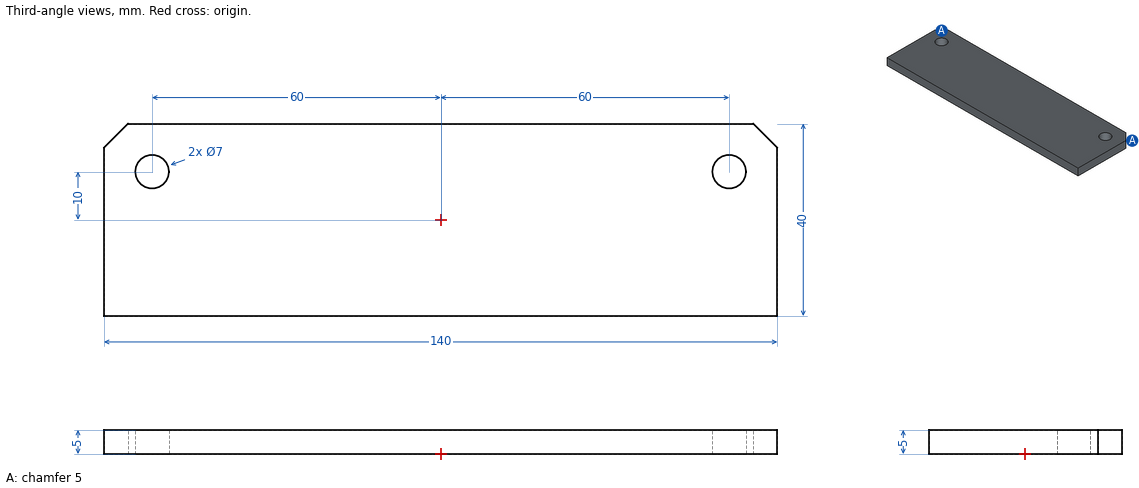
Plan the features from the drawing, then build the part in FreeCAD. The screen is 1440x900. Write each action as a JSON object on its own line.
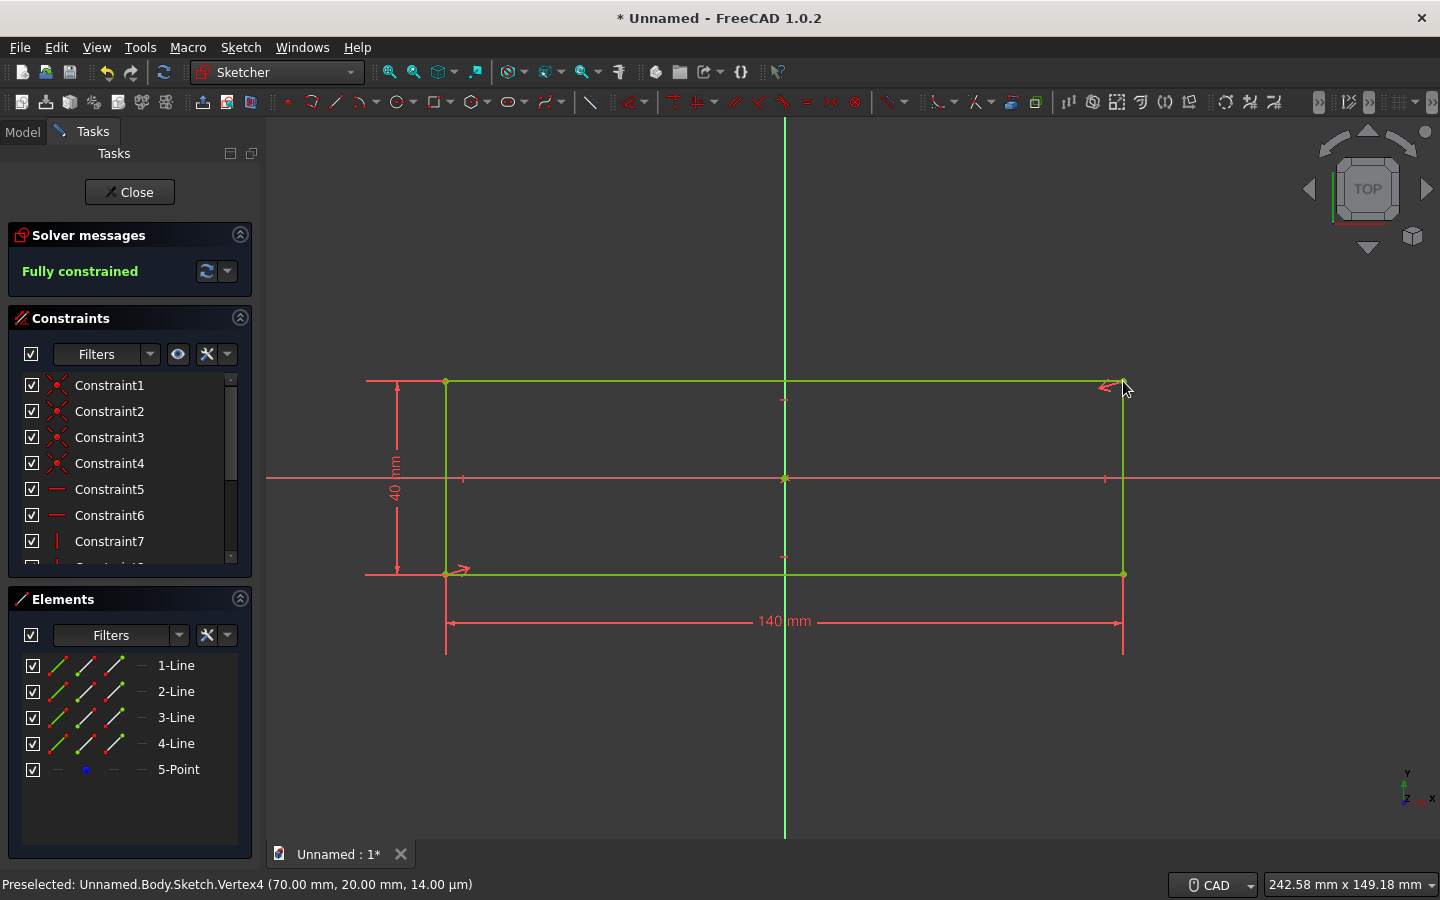
{"action": "left_click", "coordinate": [130, 192]}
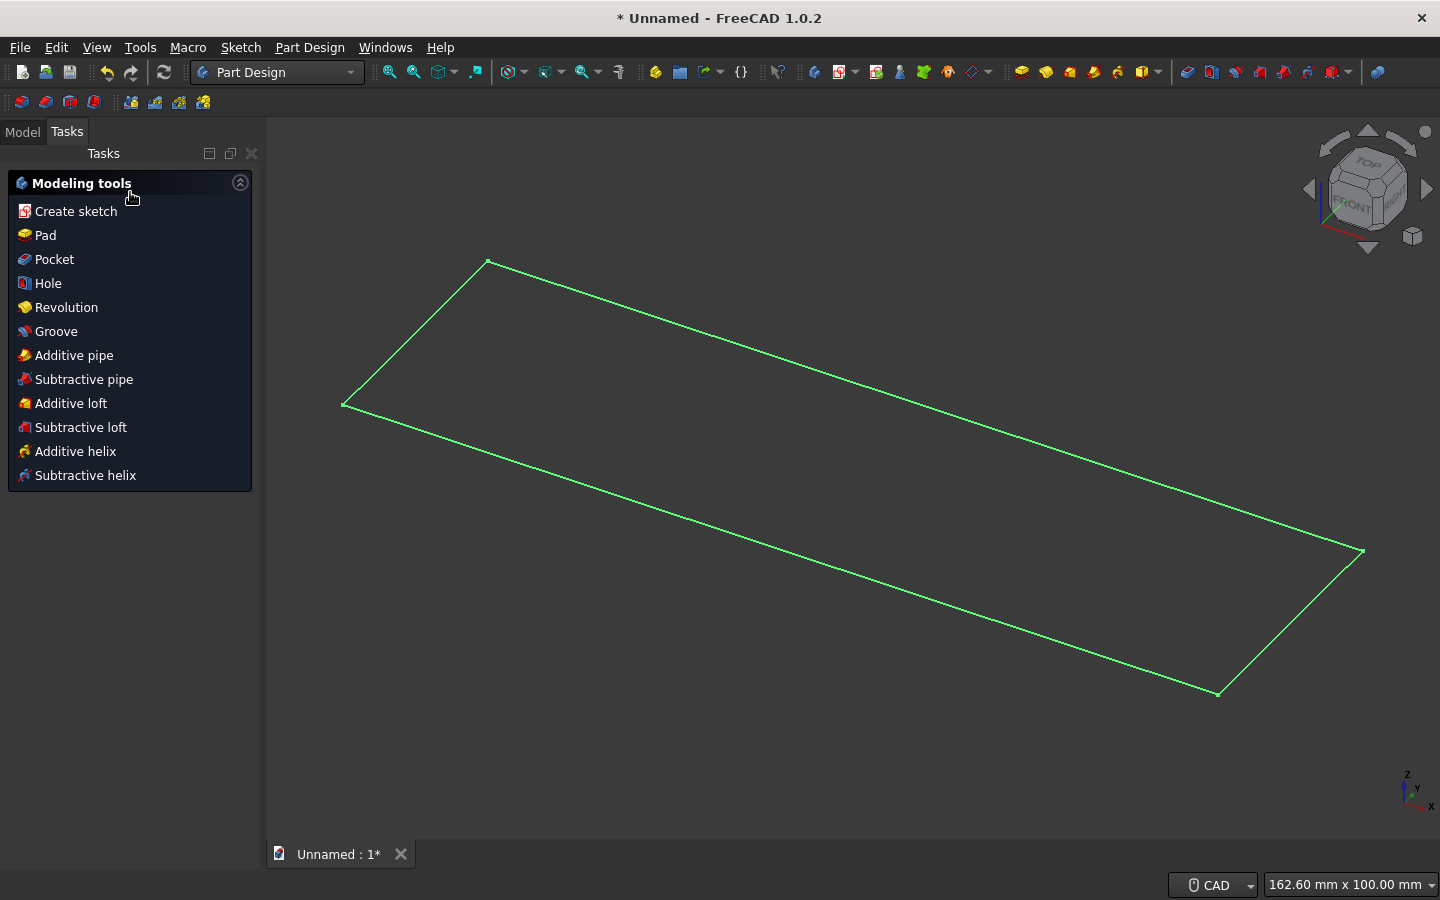
{"action": "left_click", "coordinate": [1022, 72]}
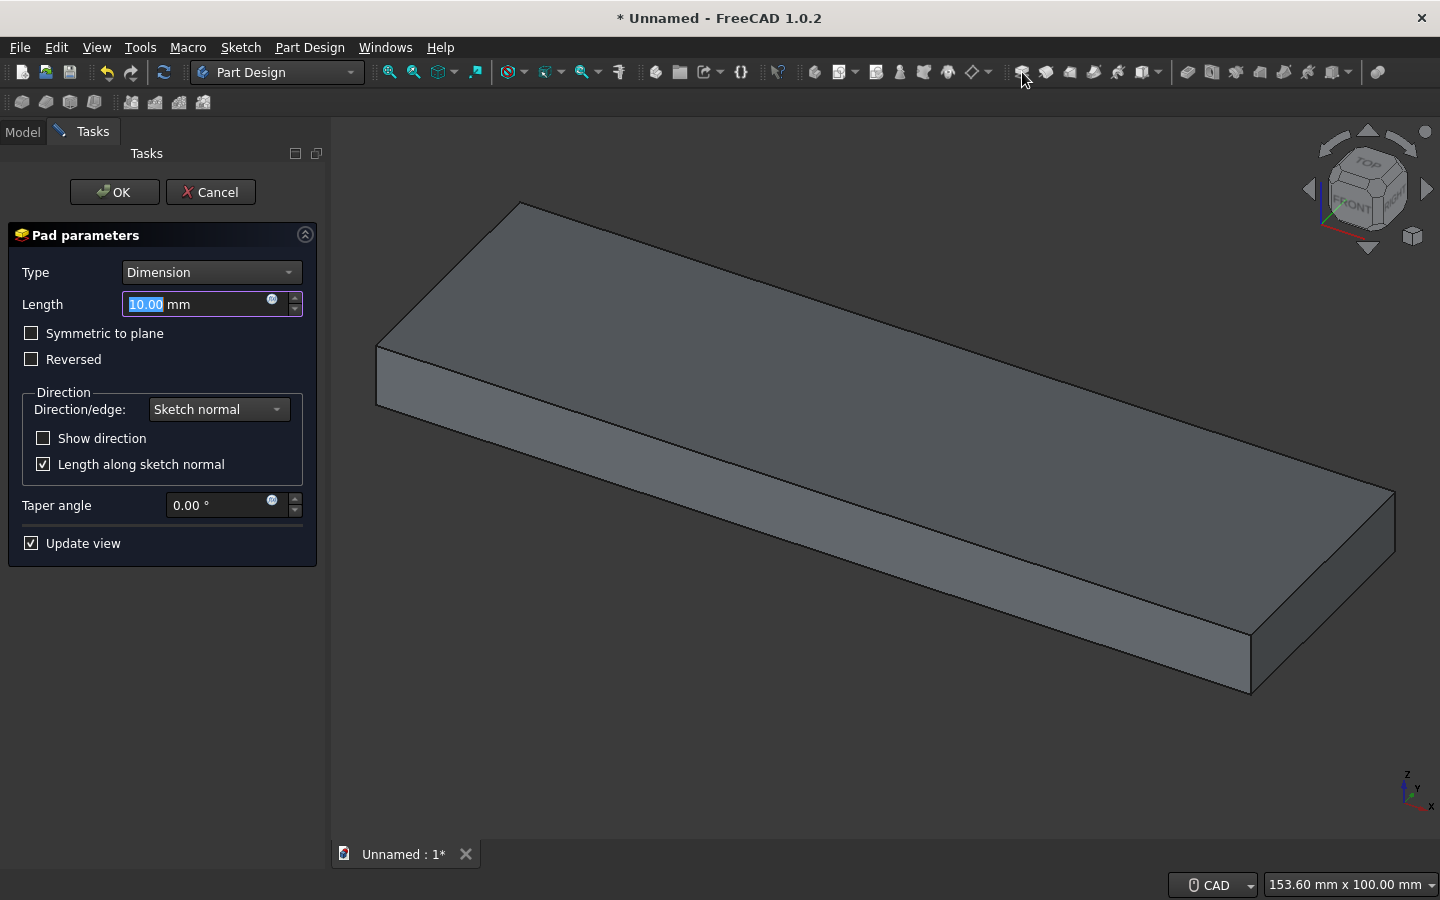
{"action": "type", "text": "5"}
{"action": "key", "text": "Tab"}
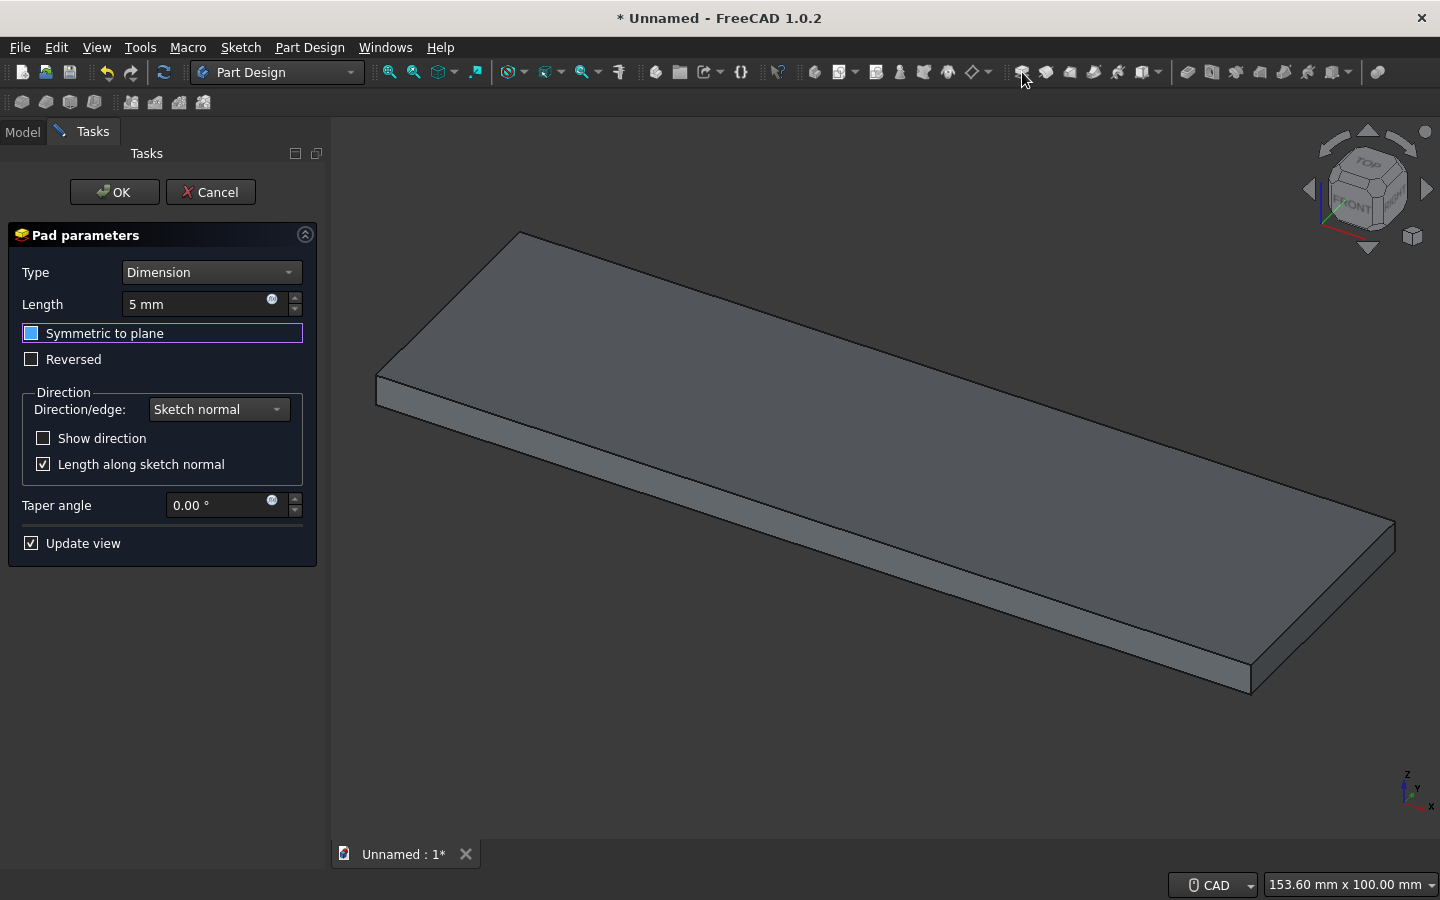
{"action": "left_click", "coordinate": [115, 192]}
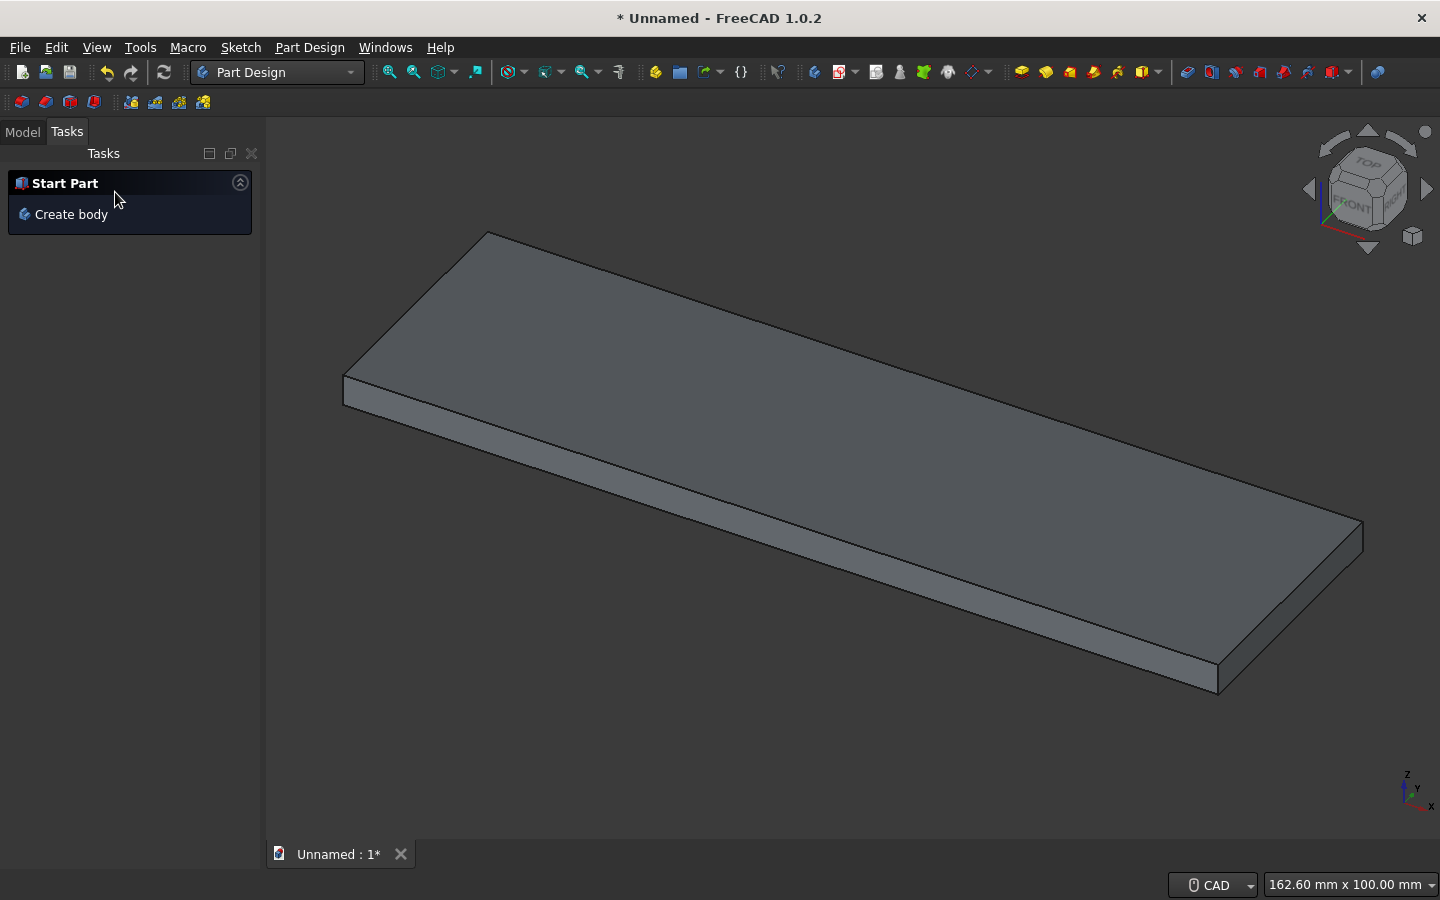
{"action": "left_click", "coordinate": [1103, 530]}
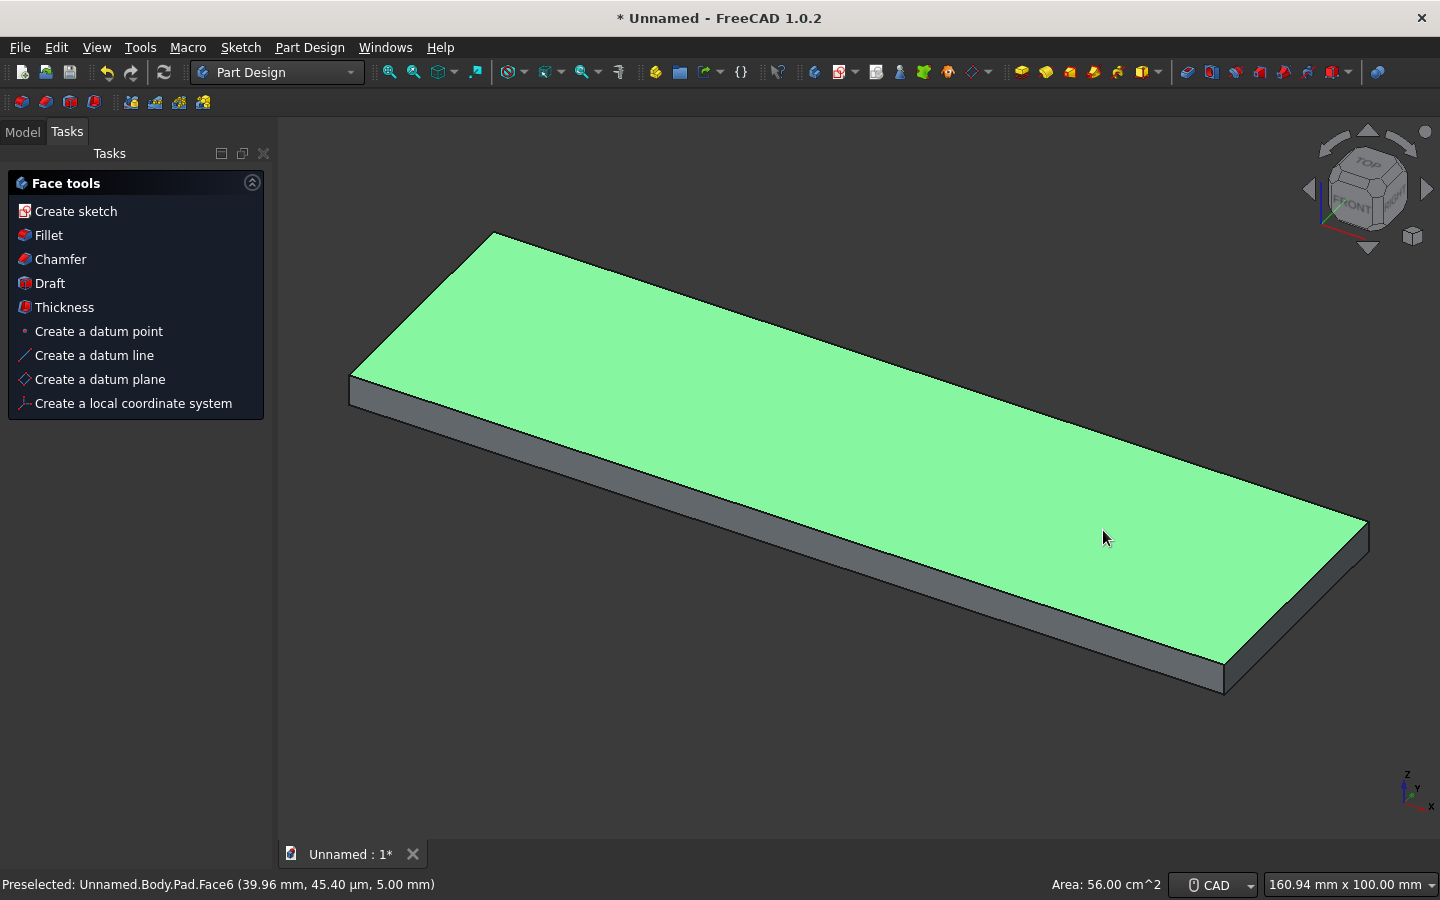
{"action": "left_click", "coordinate": [840, 72]}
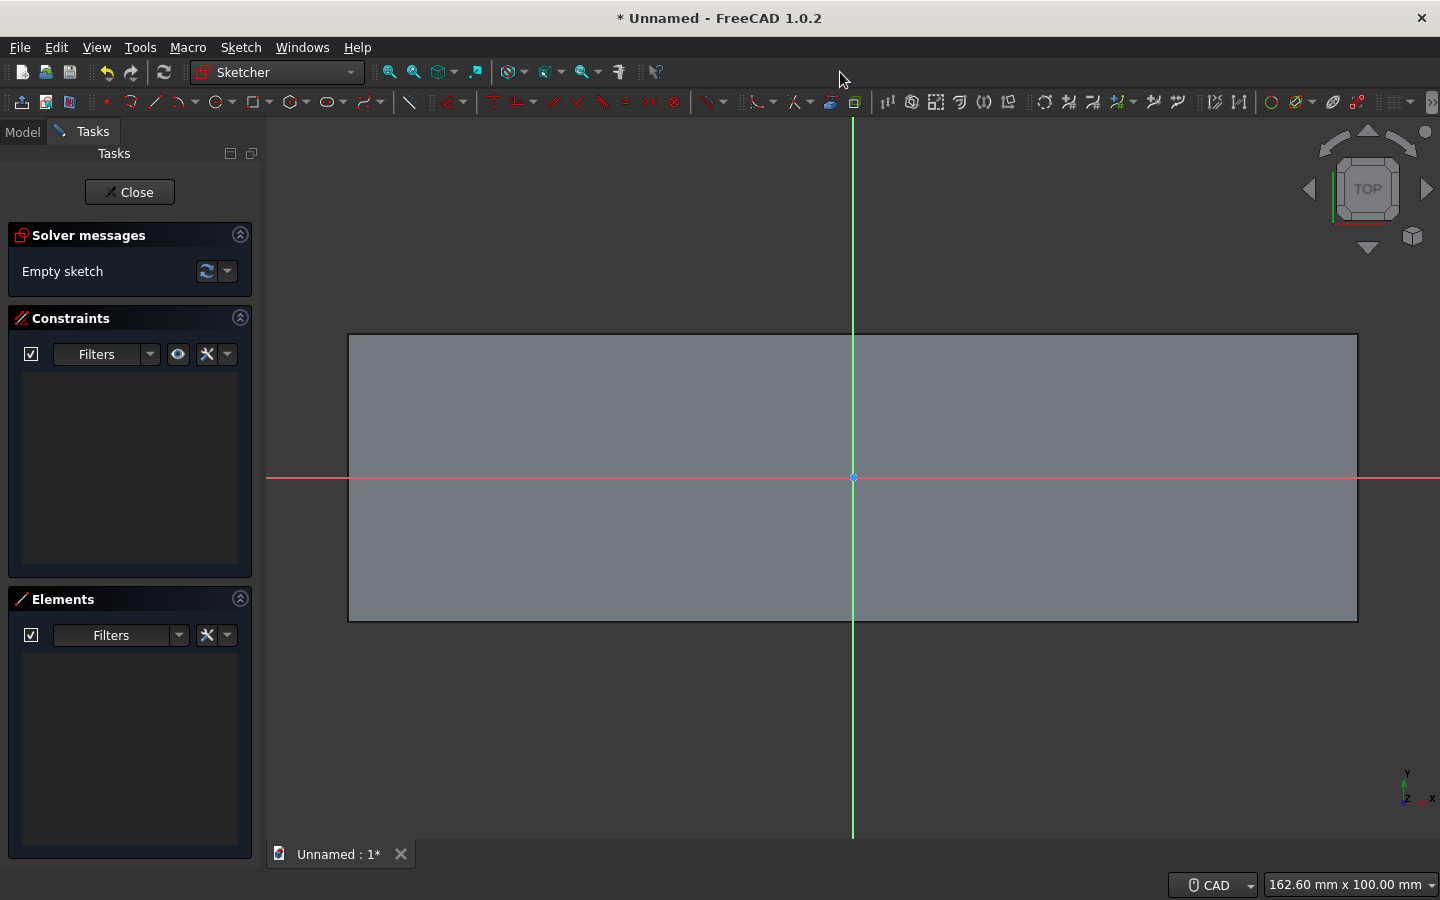
{"action": "scroll", "coordinate": [475, 698], "scroll_direction": "down", "scroll_amount": 1}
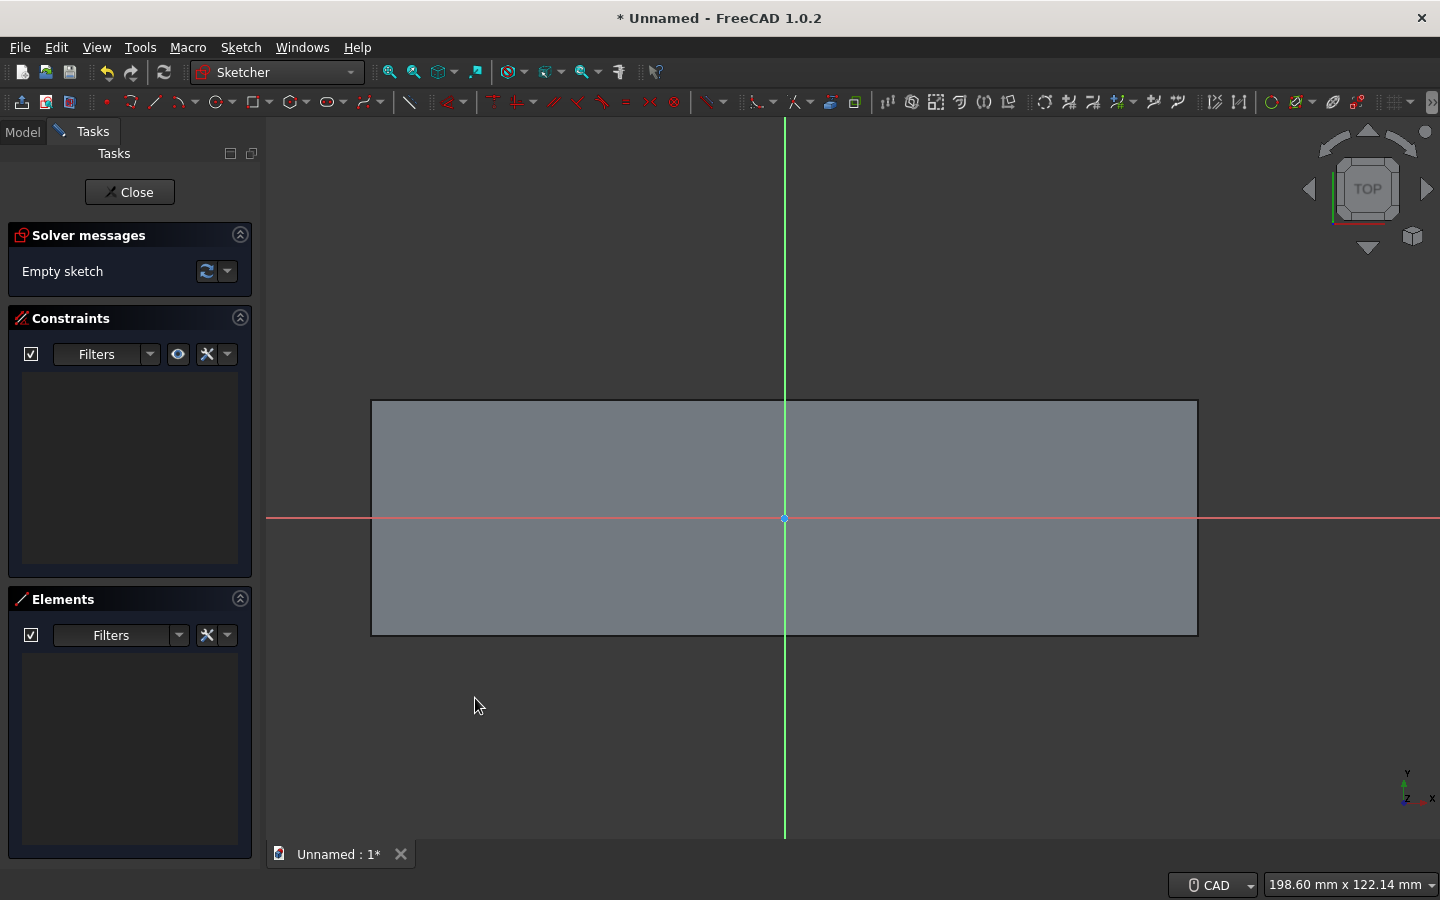
{"action": "left_click", "coordinate": [216, 102]}